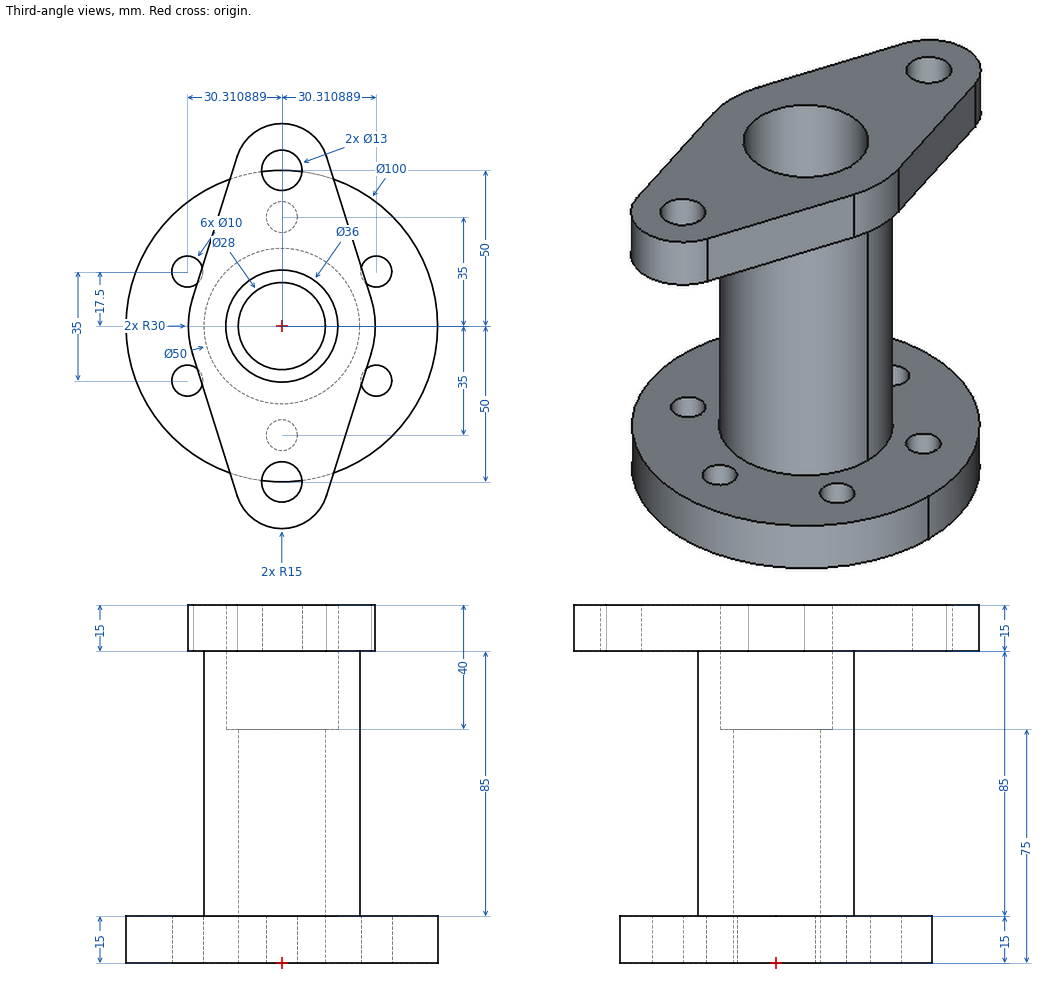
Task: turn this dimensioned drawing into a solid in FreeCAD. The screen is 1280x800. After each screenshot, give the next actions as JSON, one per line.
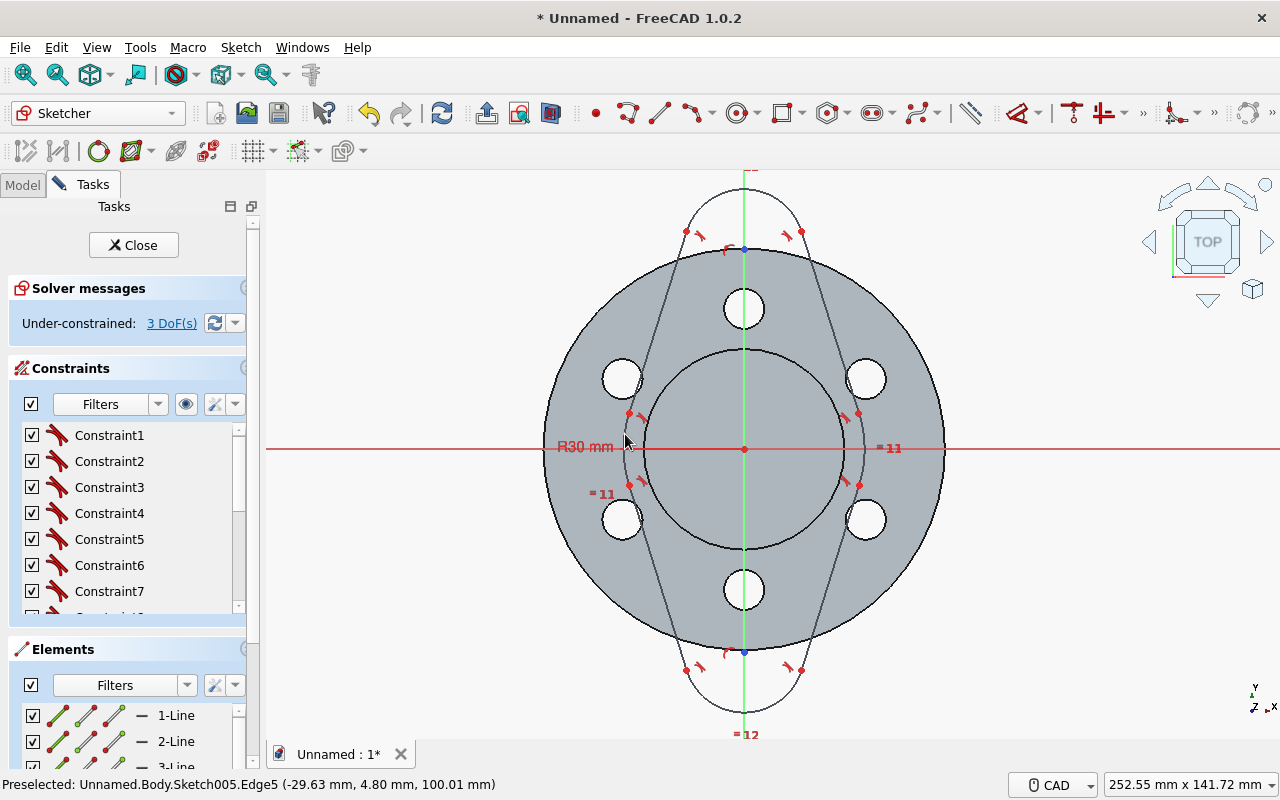
{"action": "left_click", "coordinate": [715, 705]}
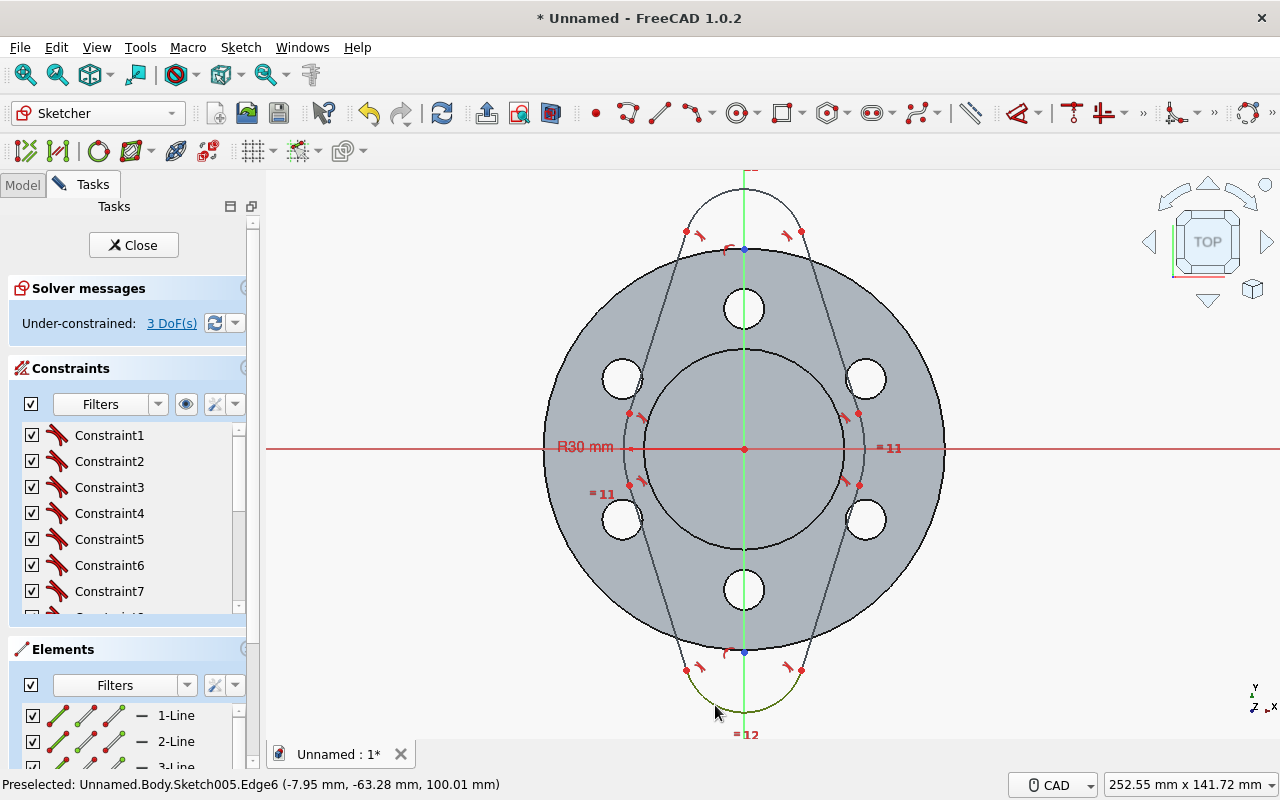
{"action": "key", "text": "k r"}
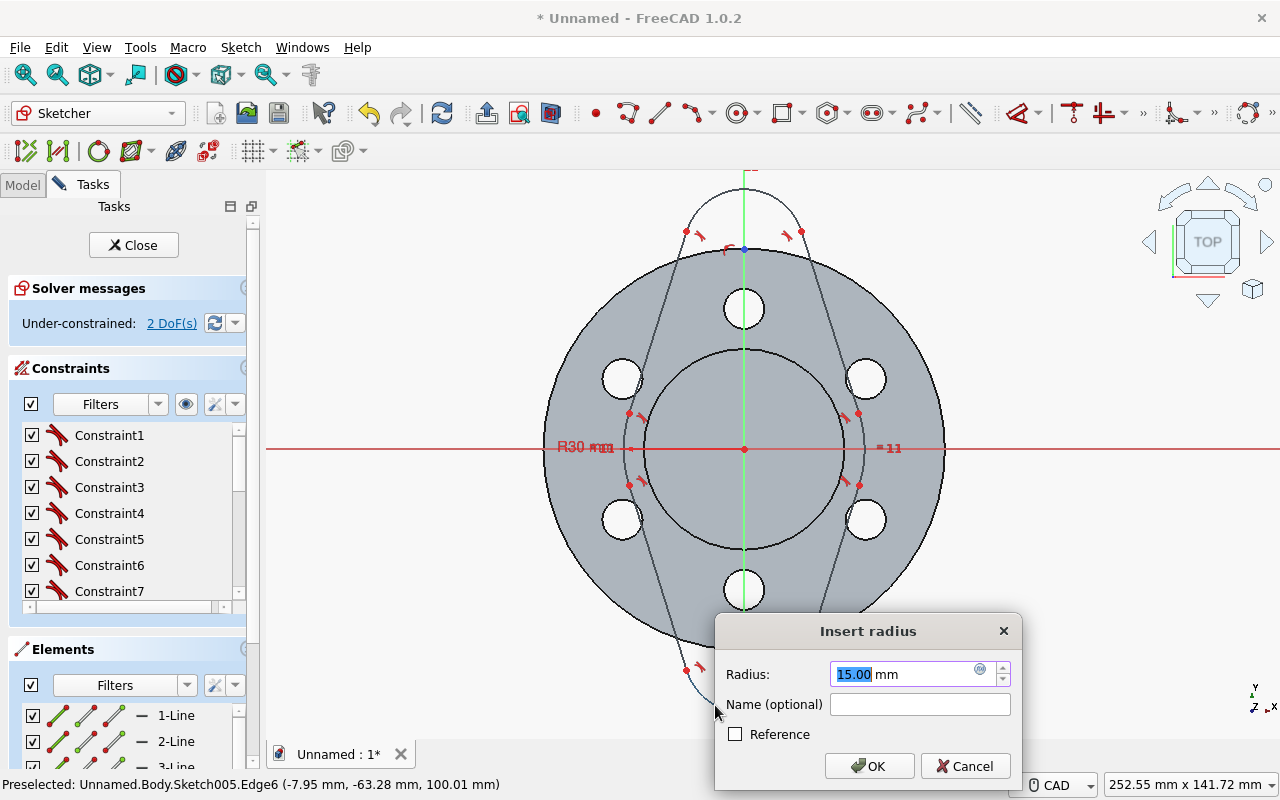
{"action": "type", "text": "15"}
{"action": "key", "text": "Return"}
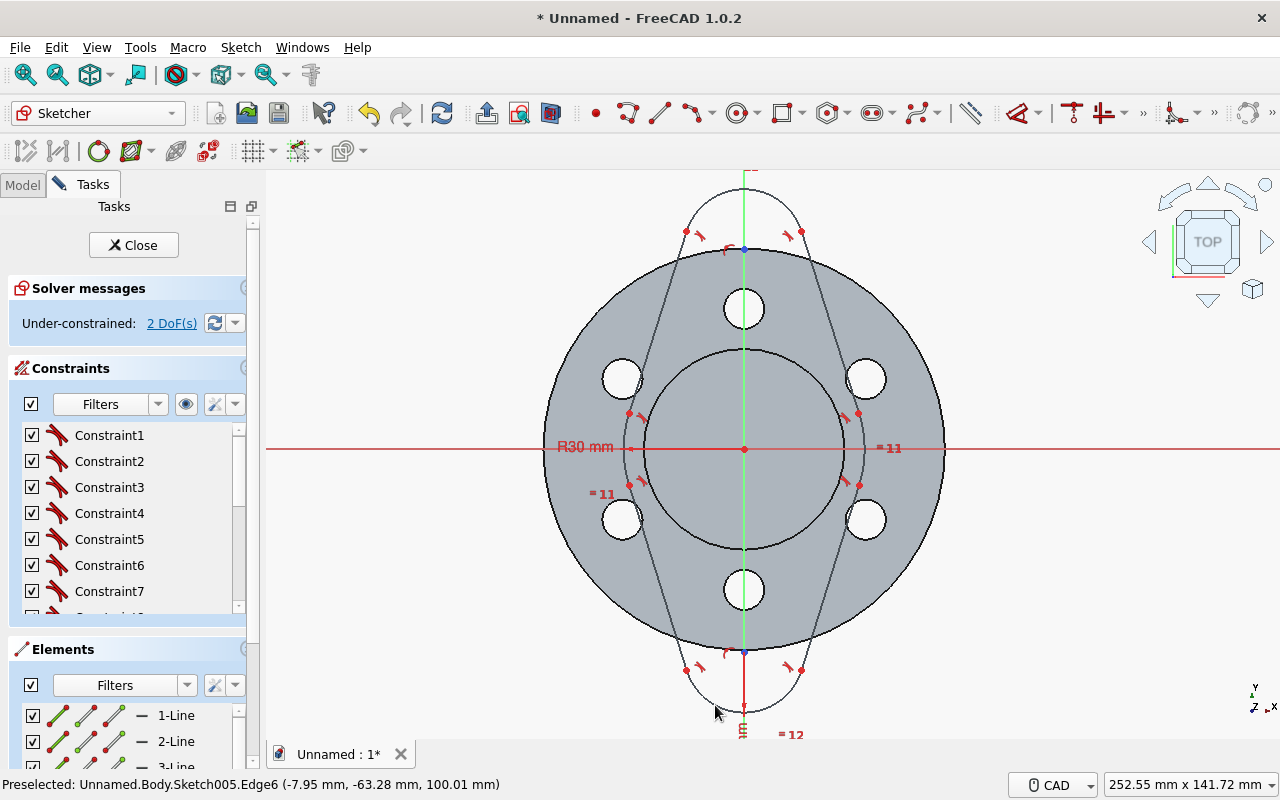
{"action": "left_click", "coordinate": [744, 652]}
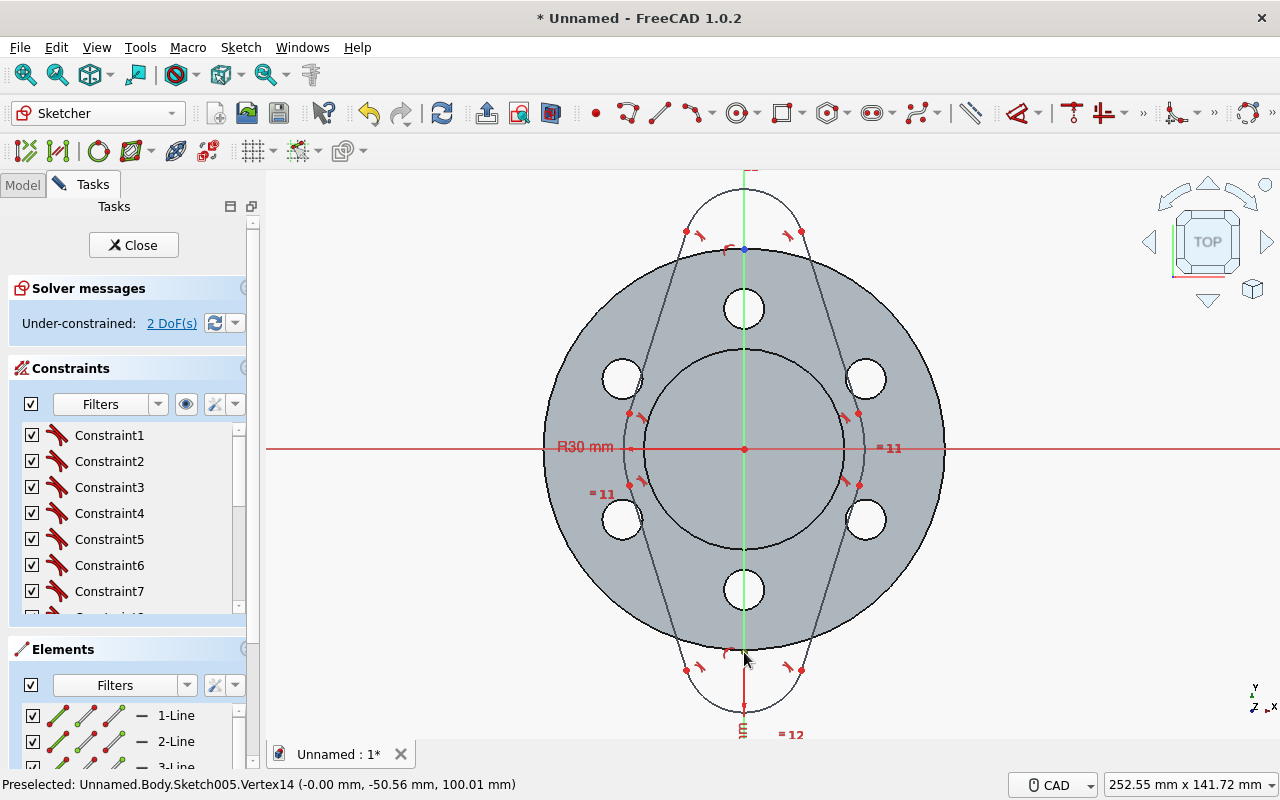
{"action": "key", "text": "i"}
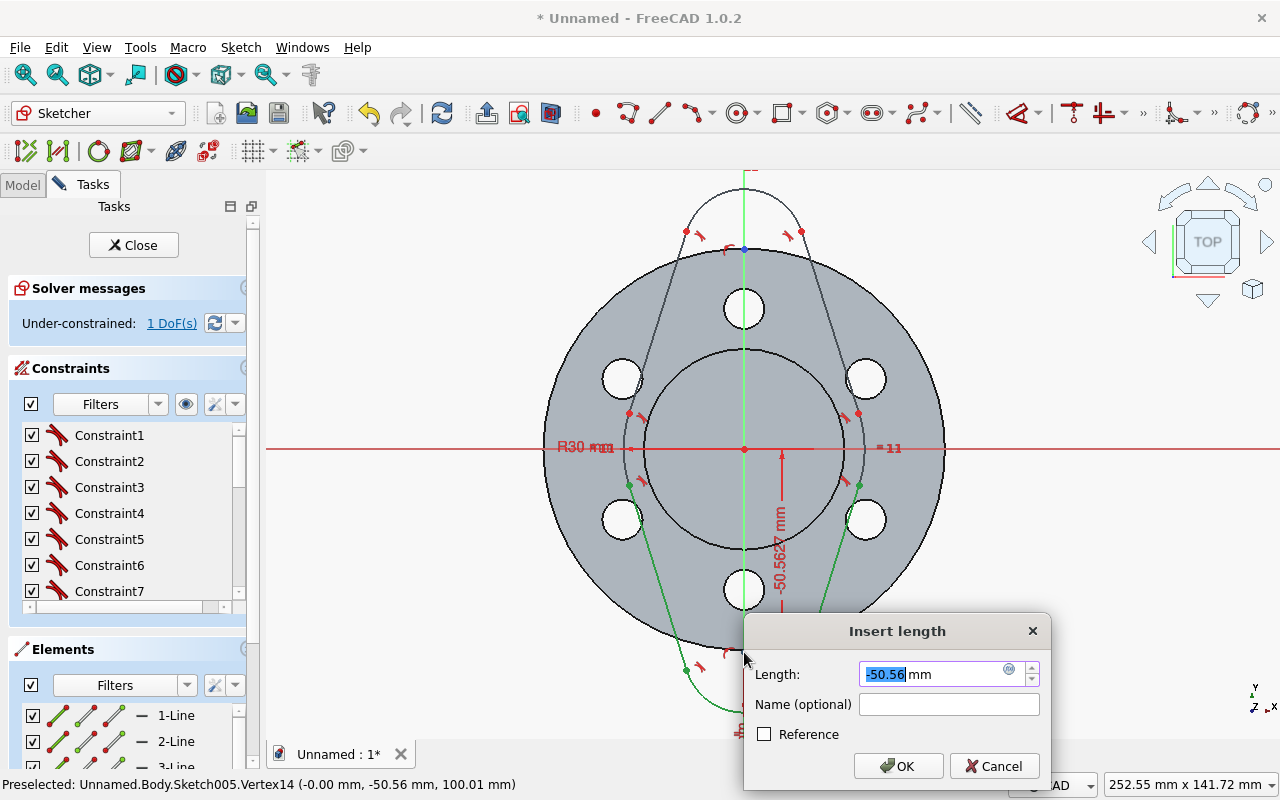
{"action": "type", "text": "-50"}
{"action": "key", "text": "Return"}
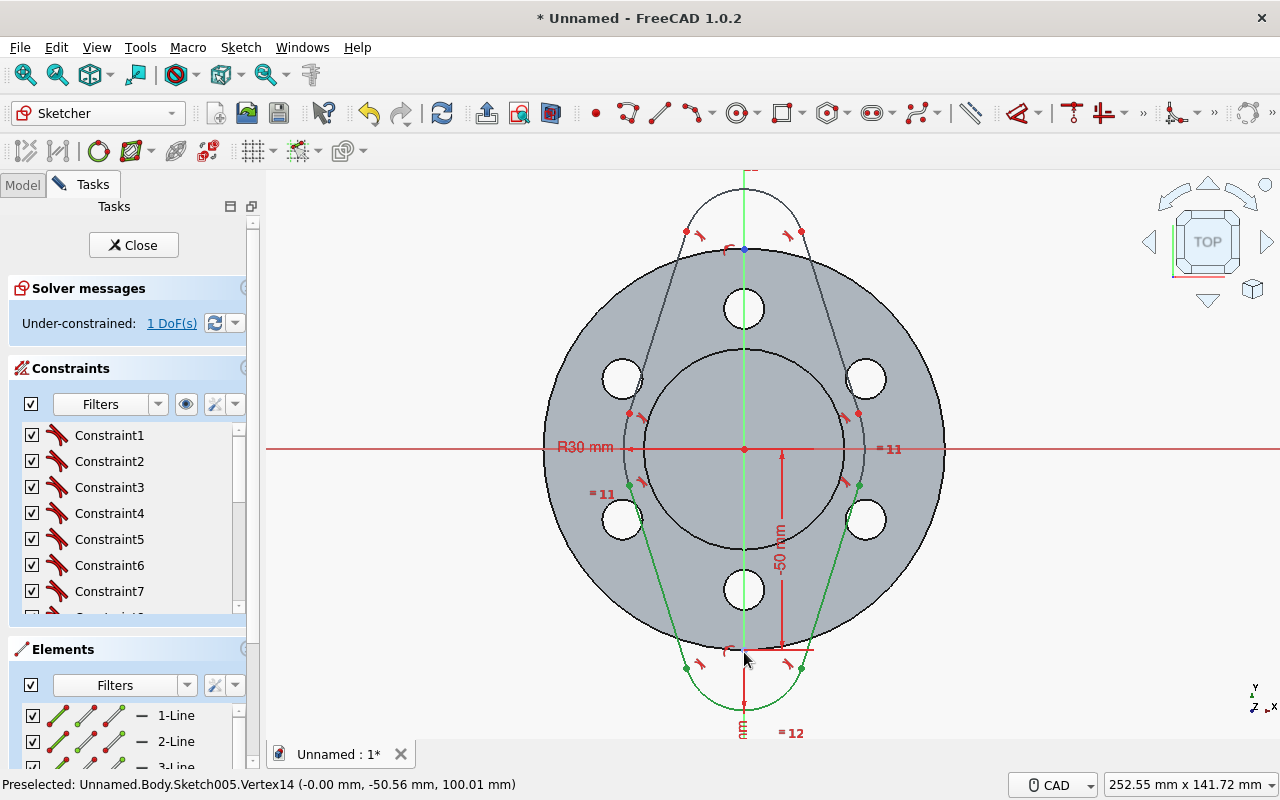
{"action": "left_click", "coordinate": [744, 249]}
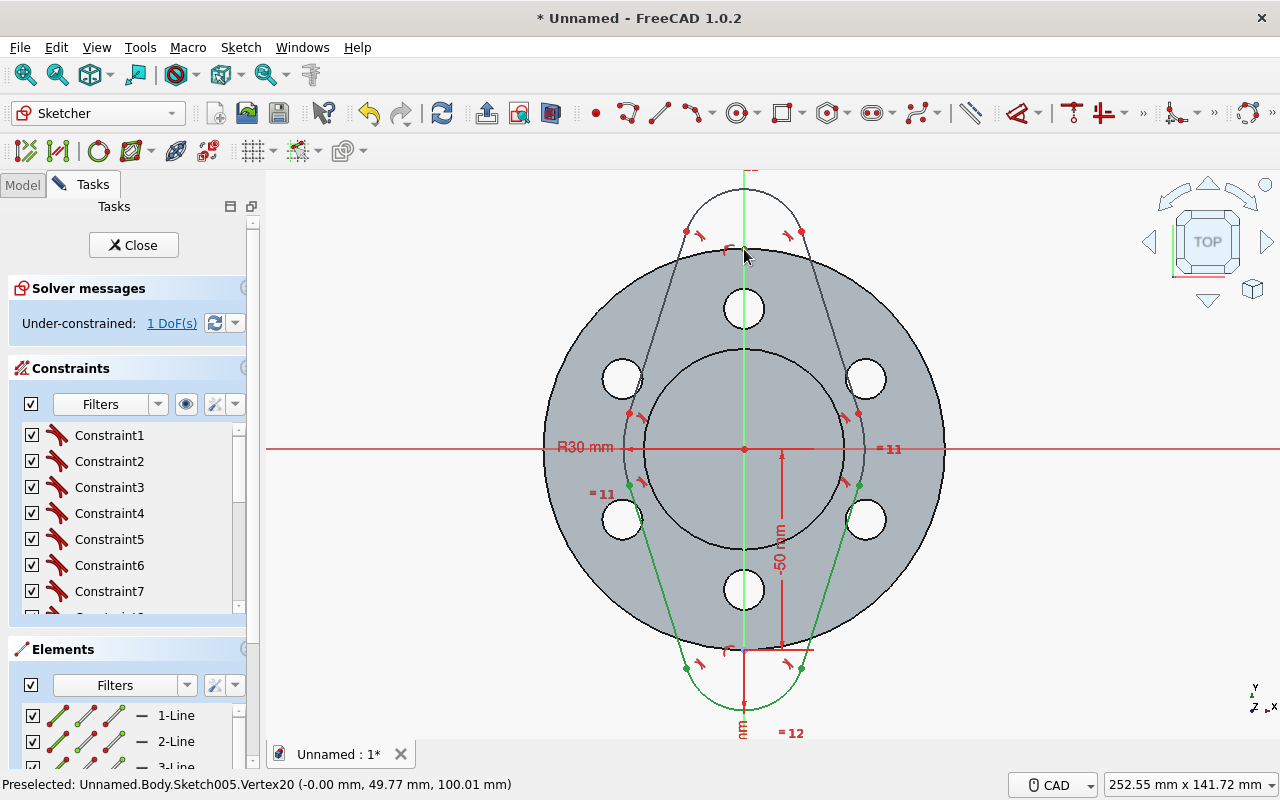
{"action": "key", "text": "i"}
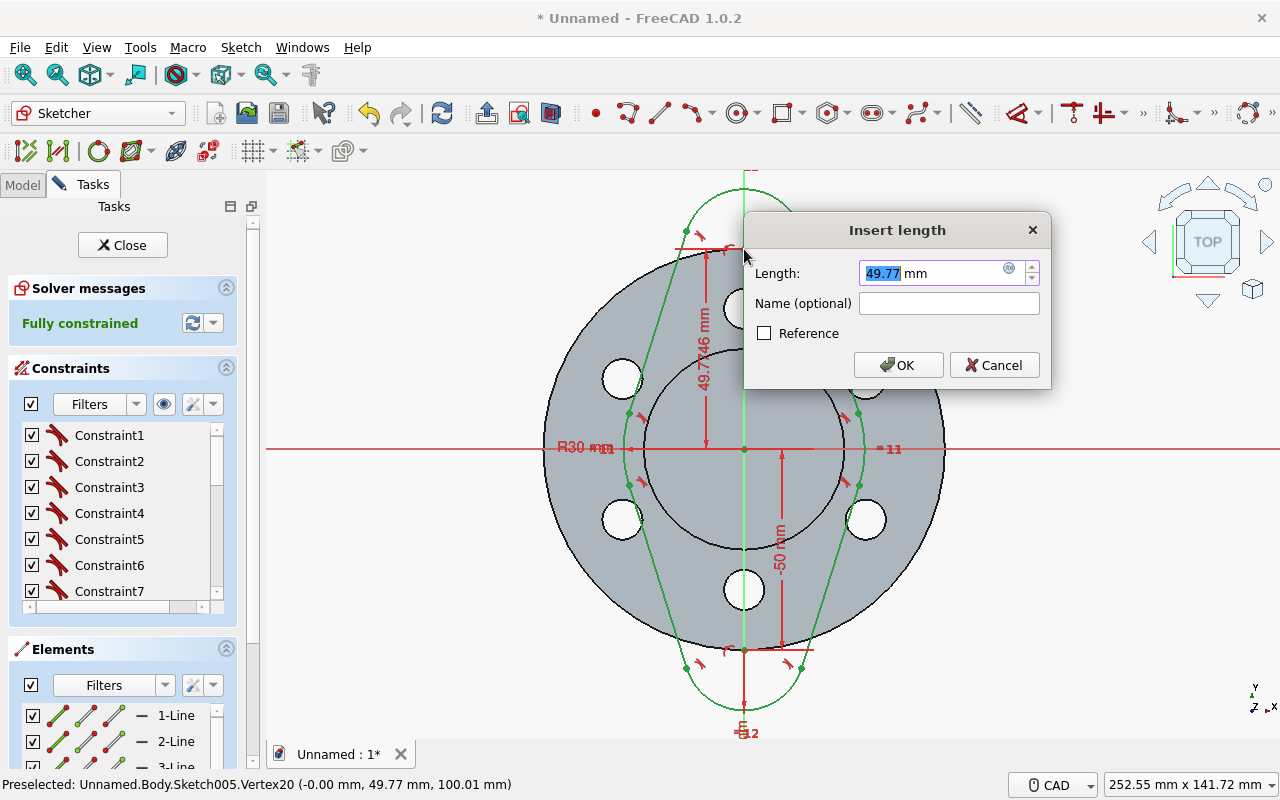
{"action": "type", "text": "50"}
{"action": "key", "text": "Return"}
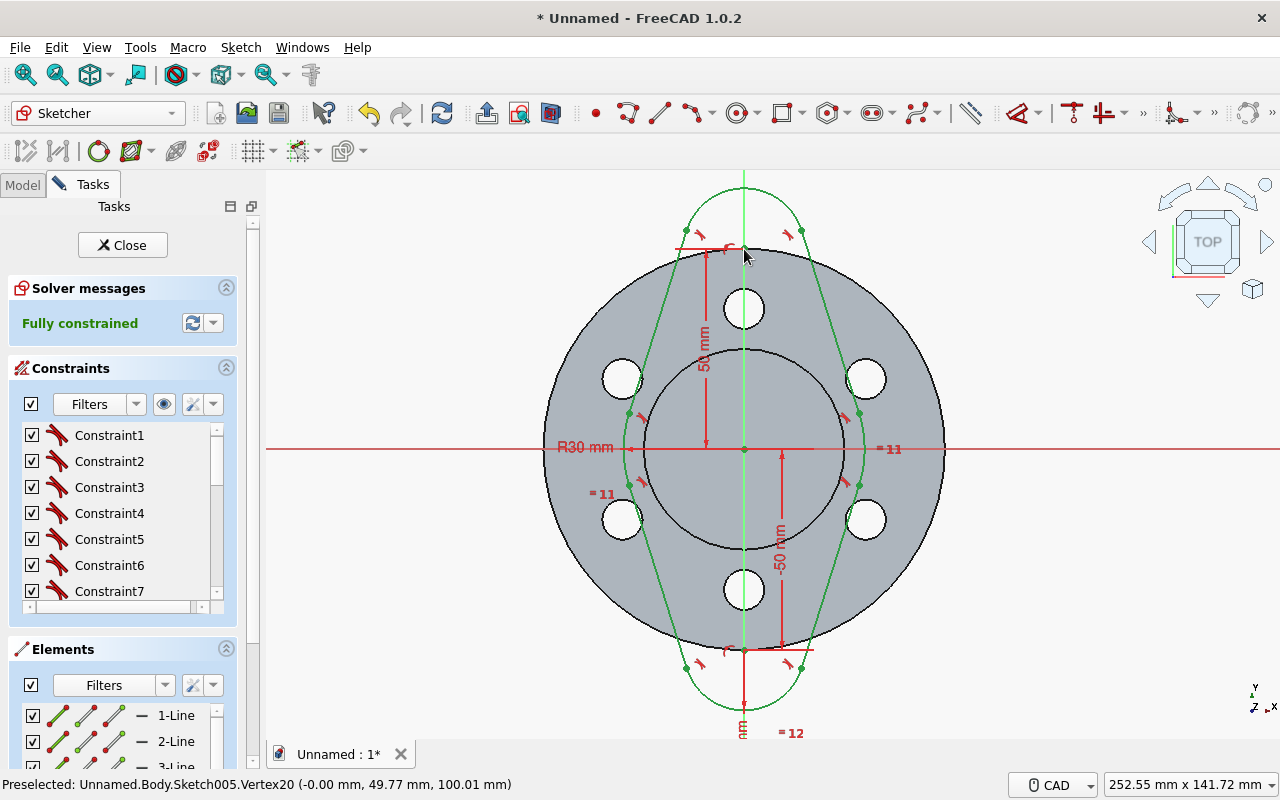
{"action": "left_click", "coordinate": [123, 245]}